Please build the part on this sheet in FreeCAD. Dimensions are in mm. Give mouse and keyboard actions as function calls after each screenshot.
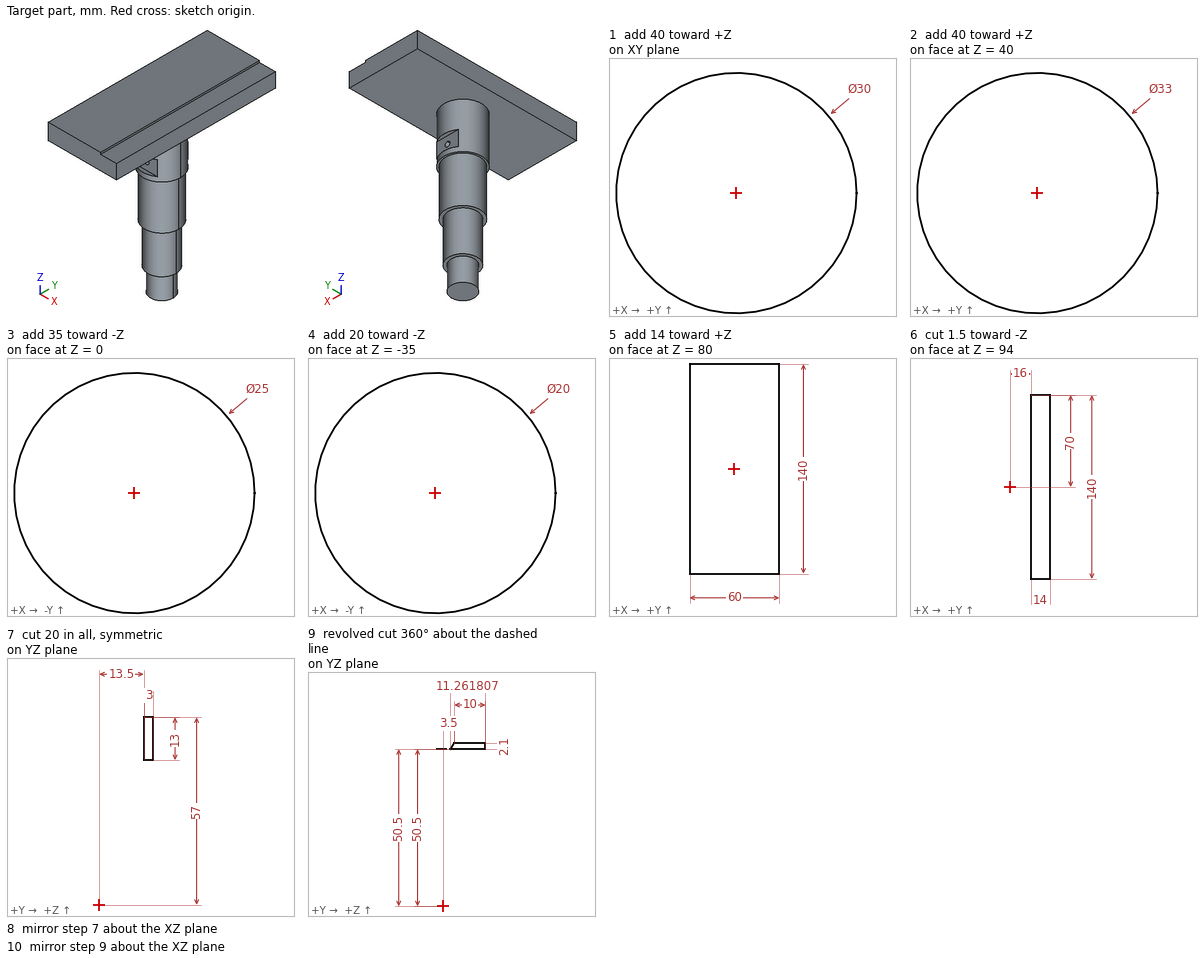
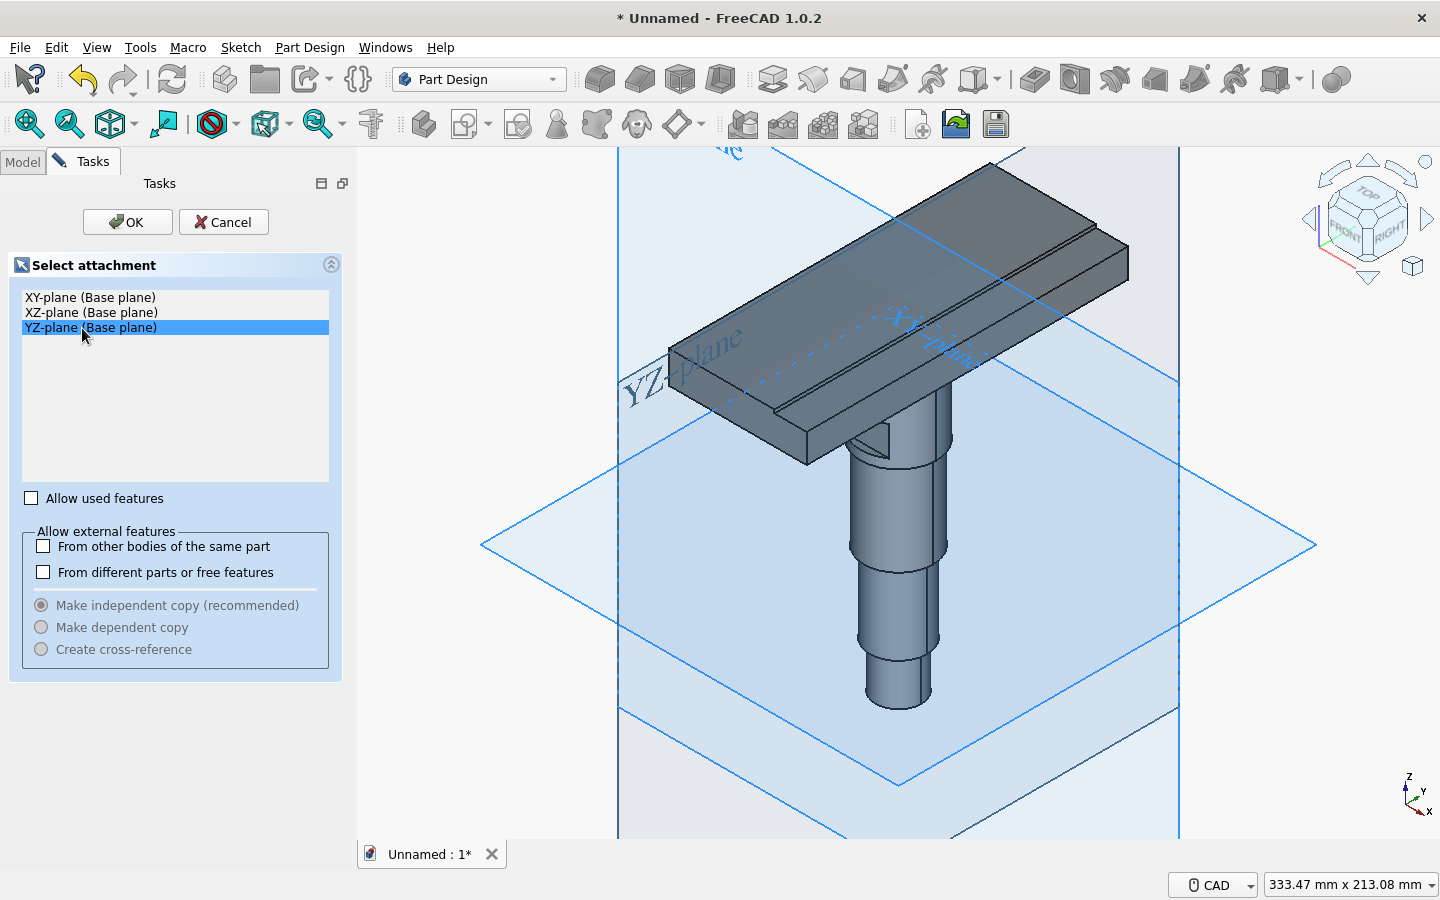
click(128, 222)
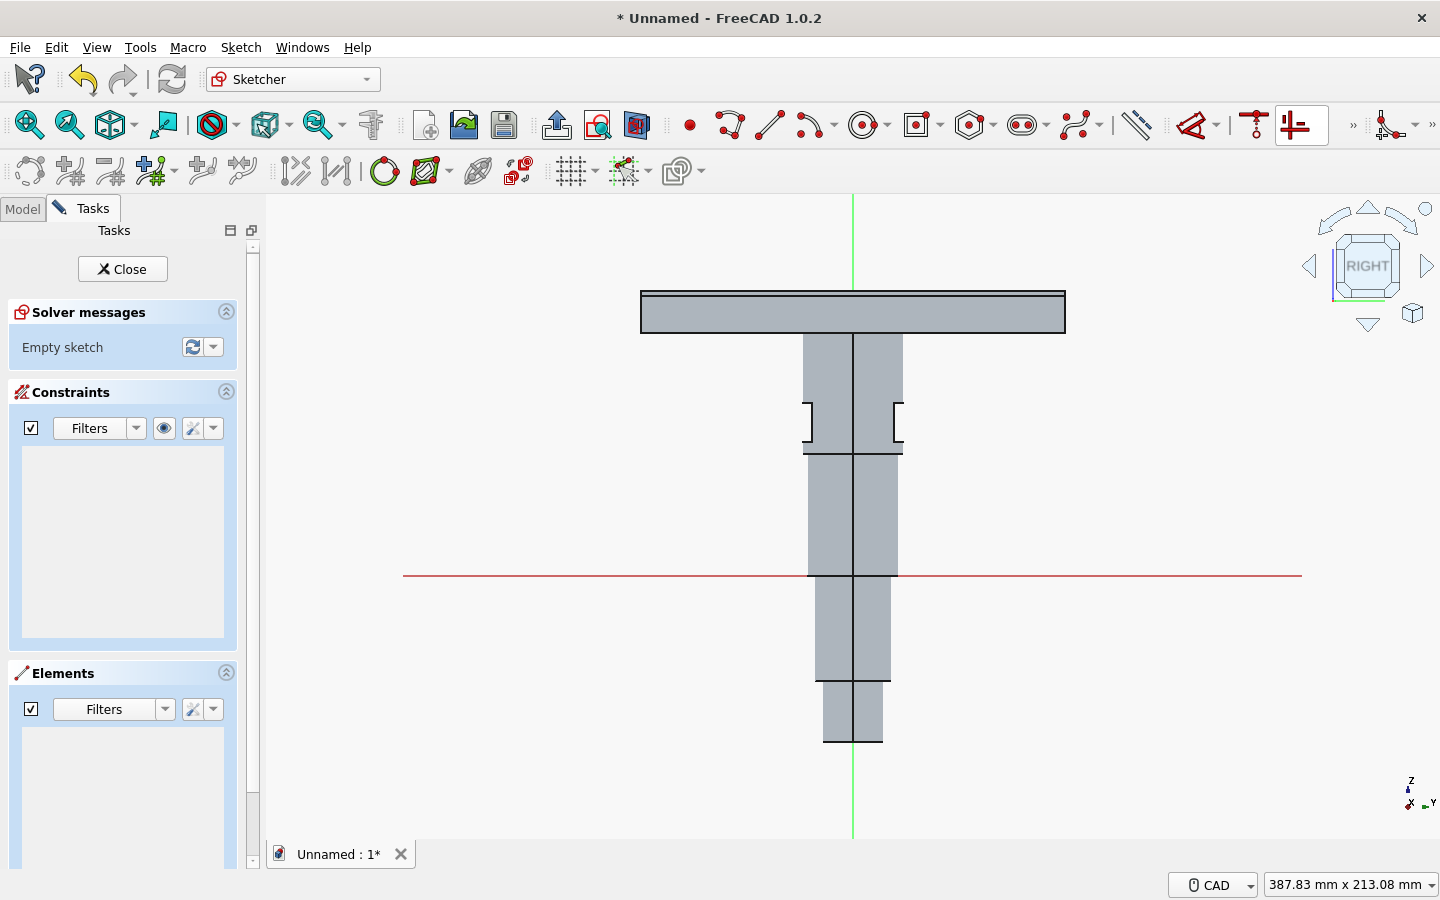
click(638, 126)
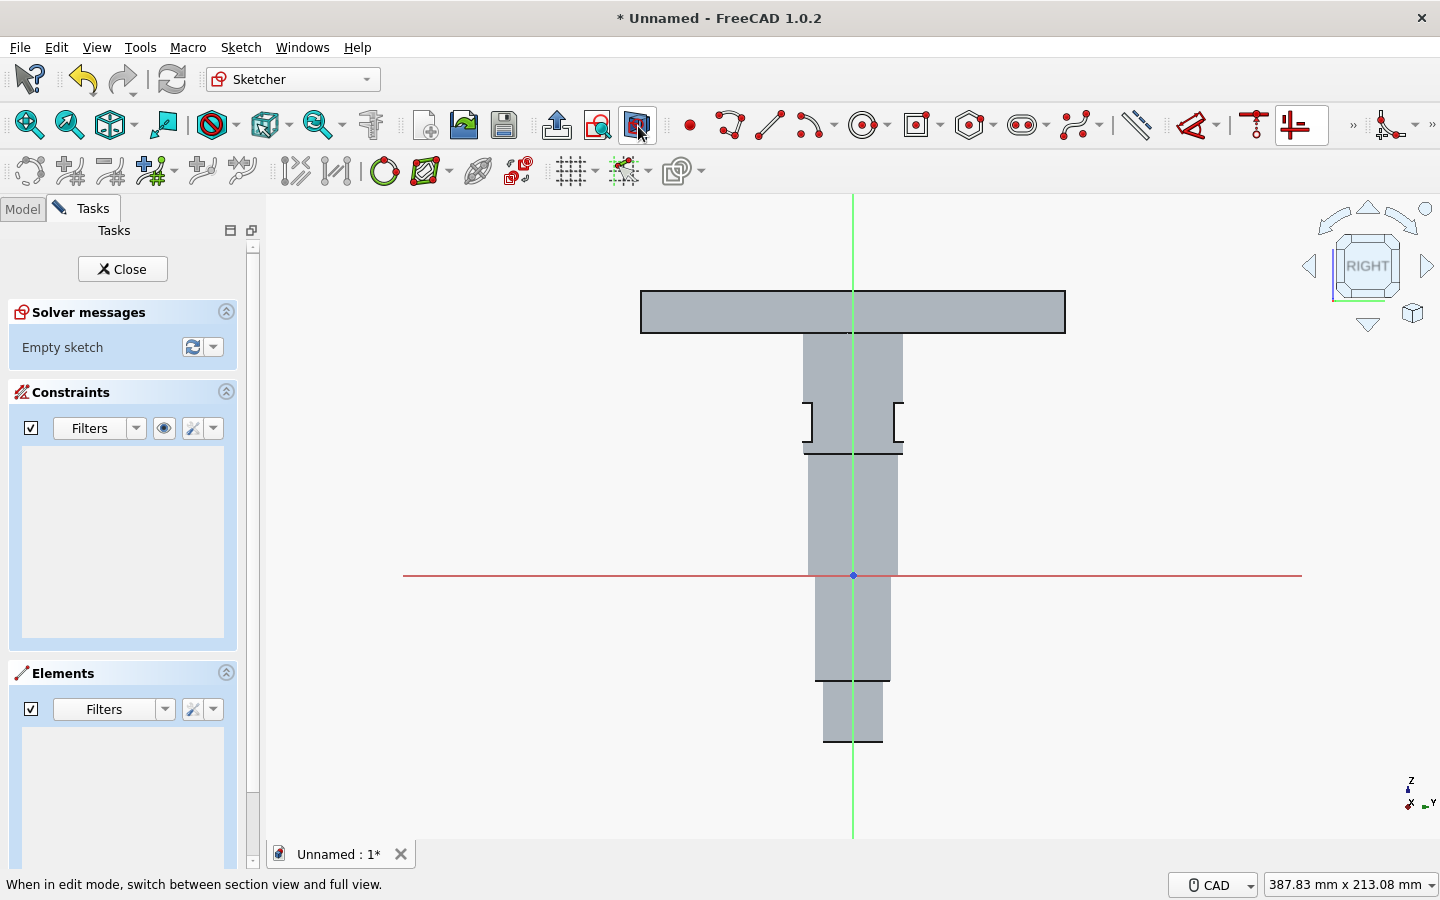
scroll(877, 412, up, 13)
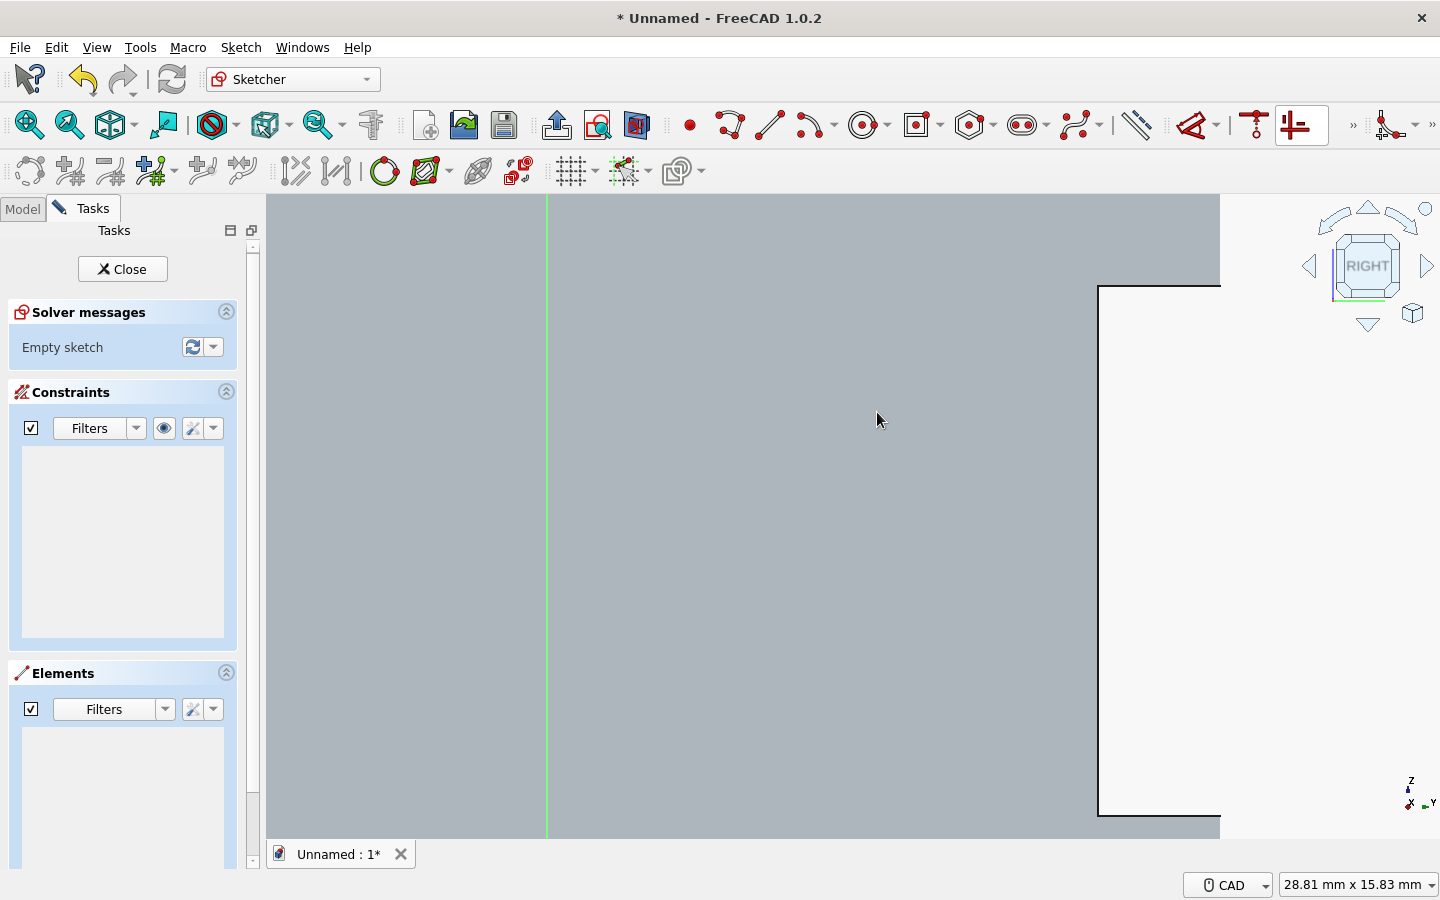
click(730, 126)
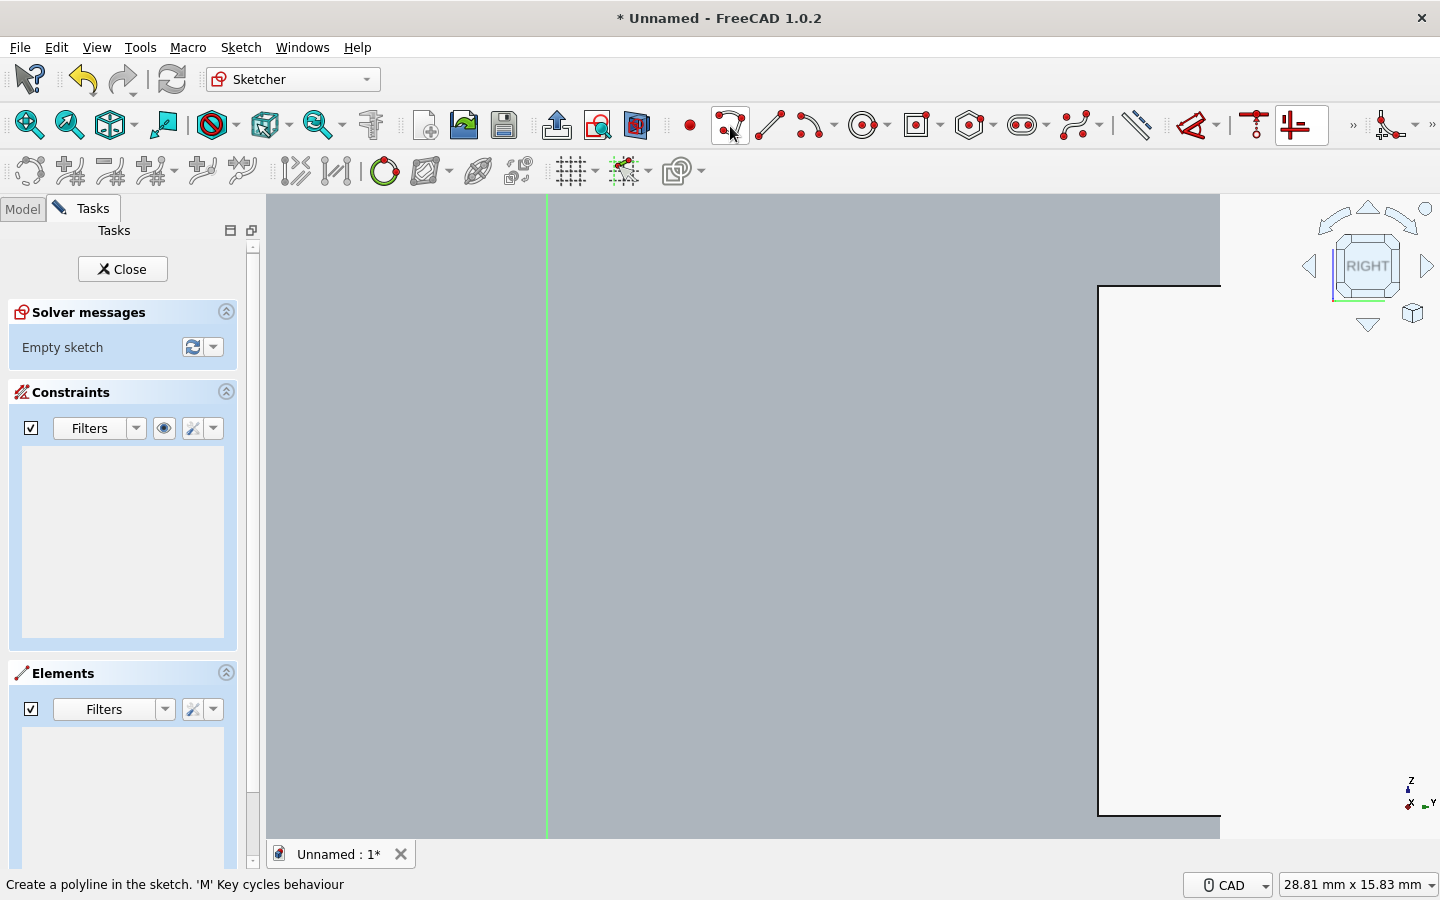
click(639, 551)
click(1098, 551)
click(1098, 466)
click(690, 466)
click(639, 552)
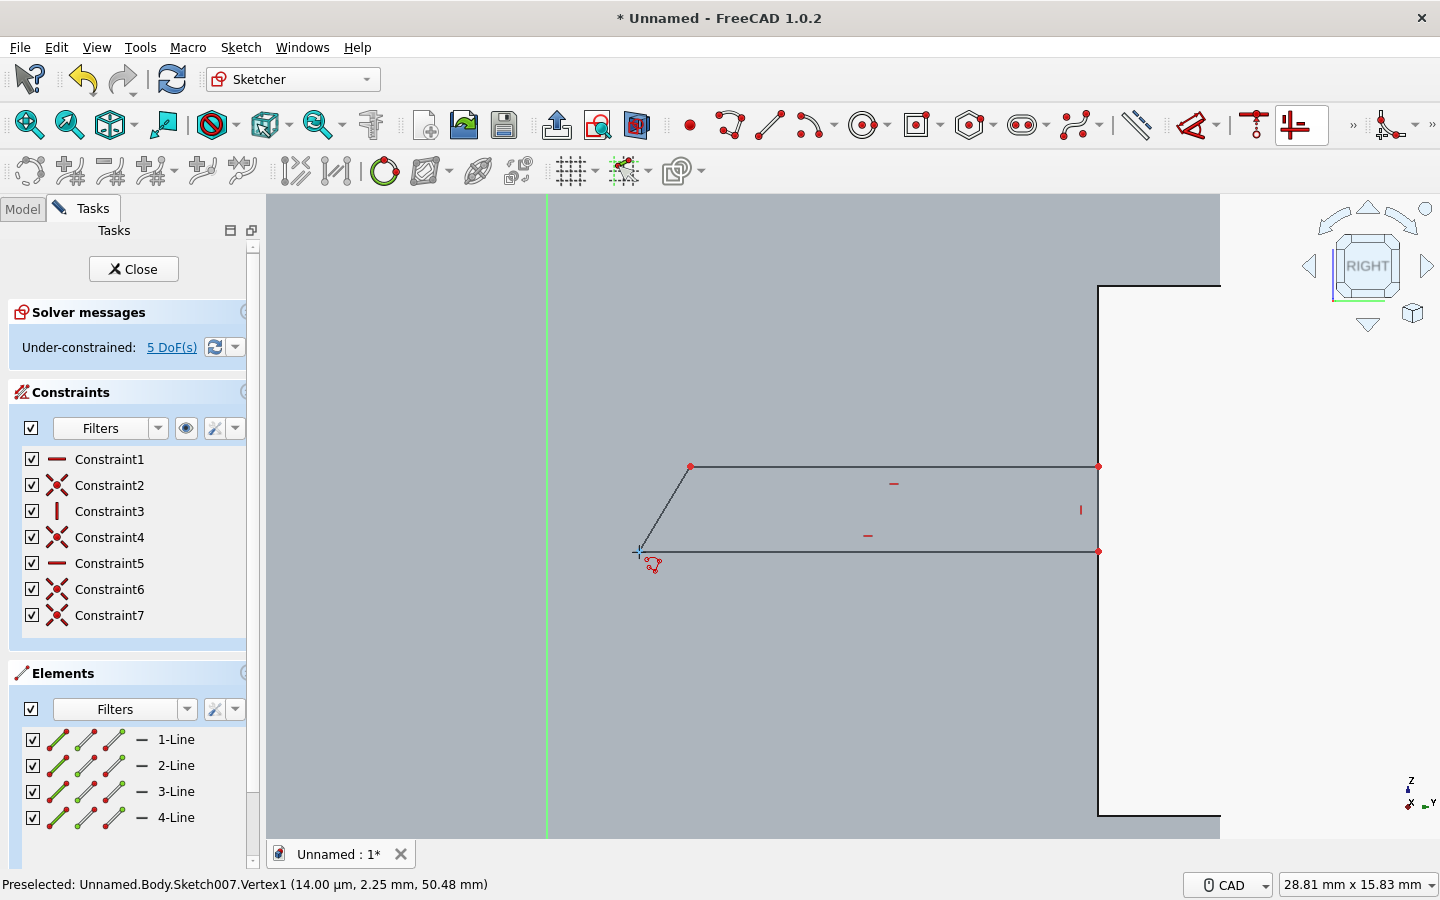
click(770, 126)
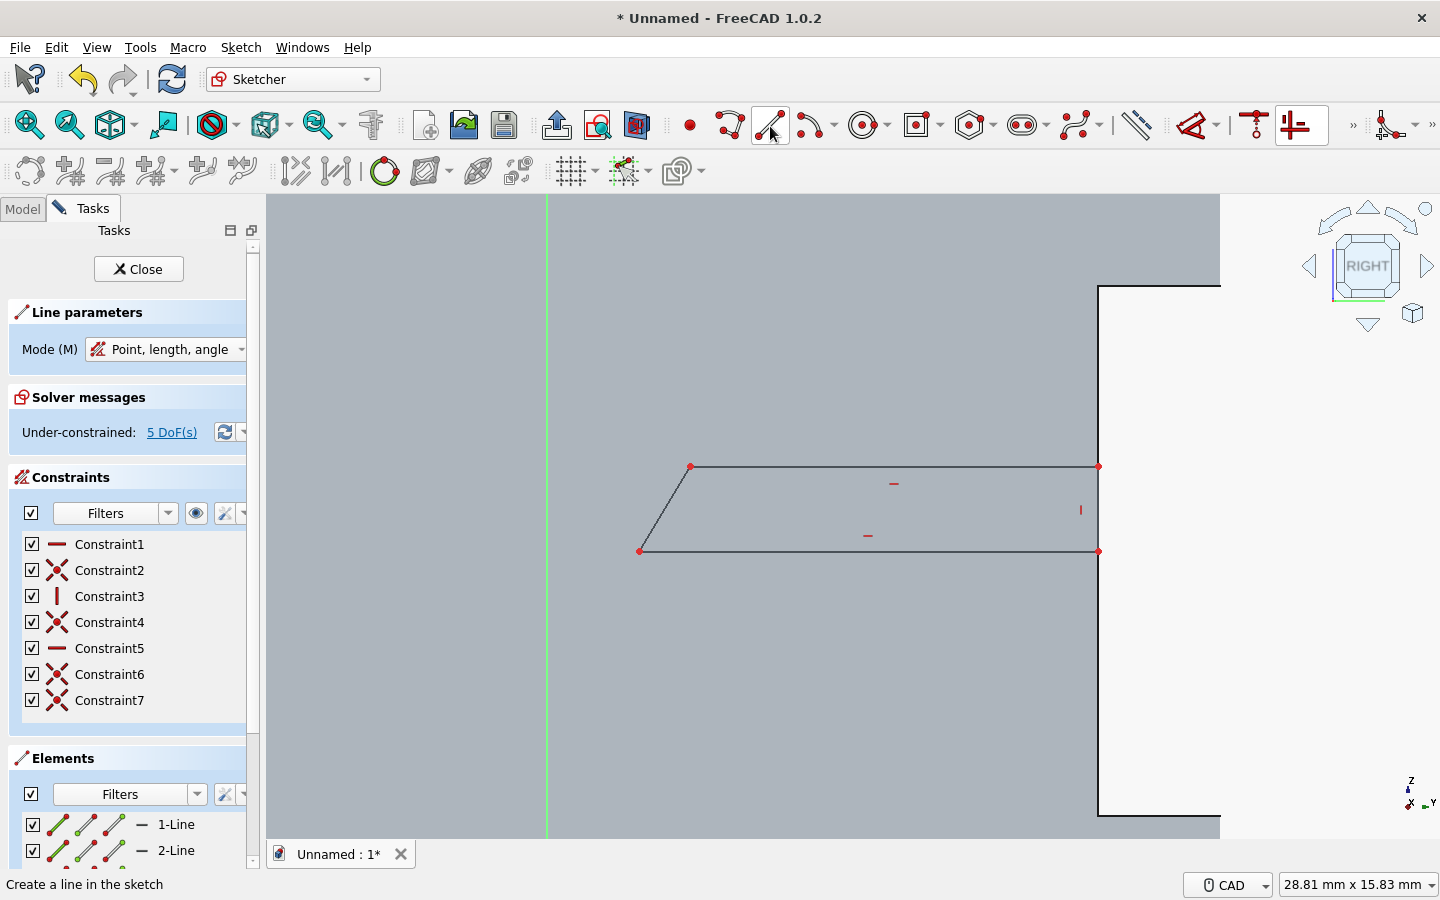
click(593, 551)
click(455, 551)
key(Escape)